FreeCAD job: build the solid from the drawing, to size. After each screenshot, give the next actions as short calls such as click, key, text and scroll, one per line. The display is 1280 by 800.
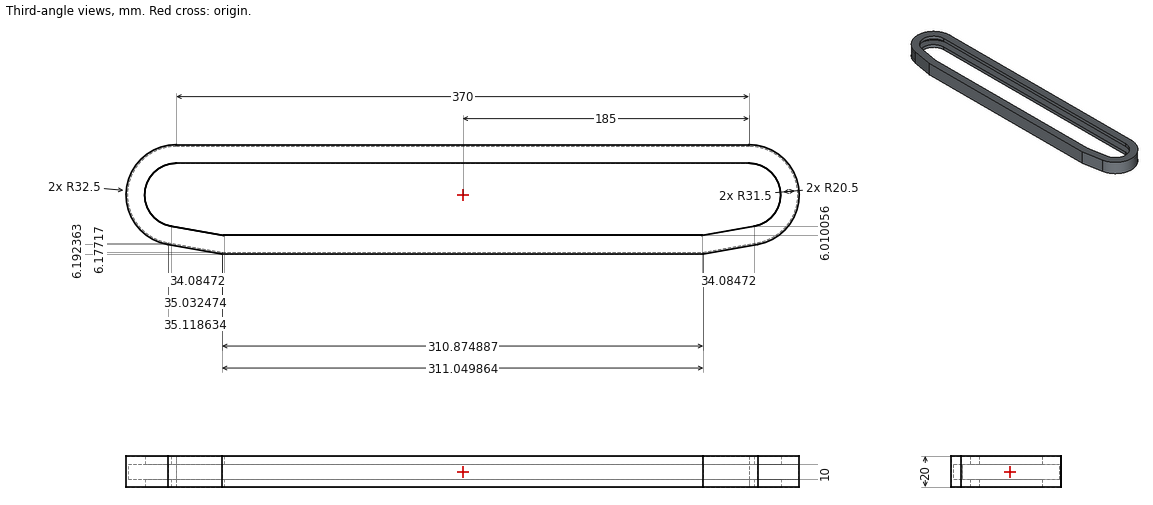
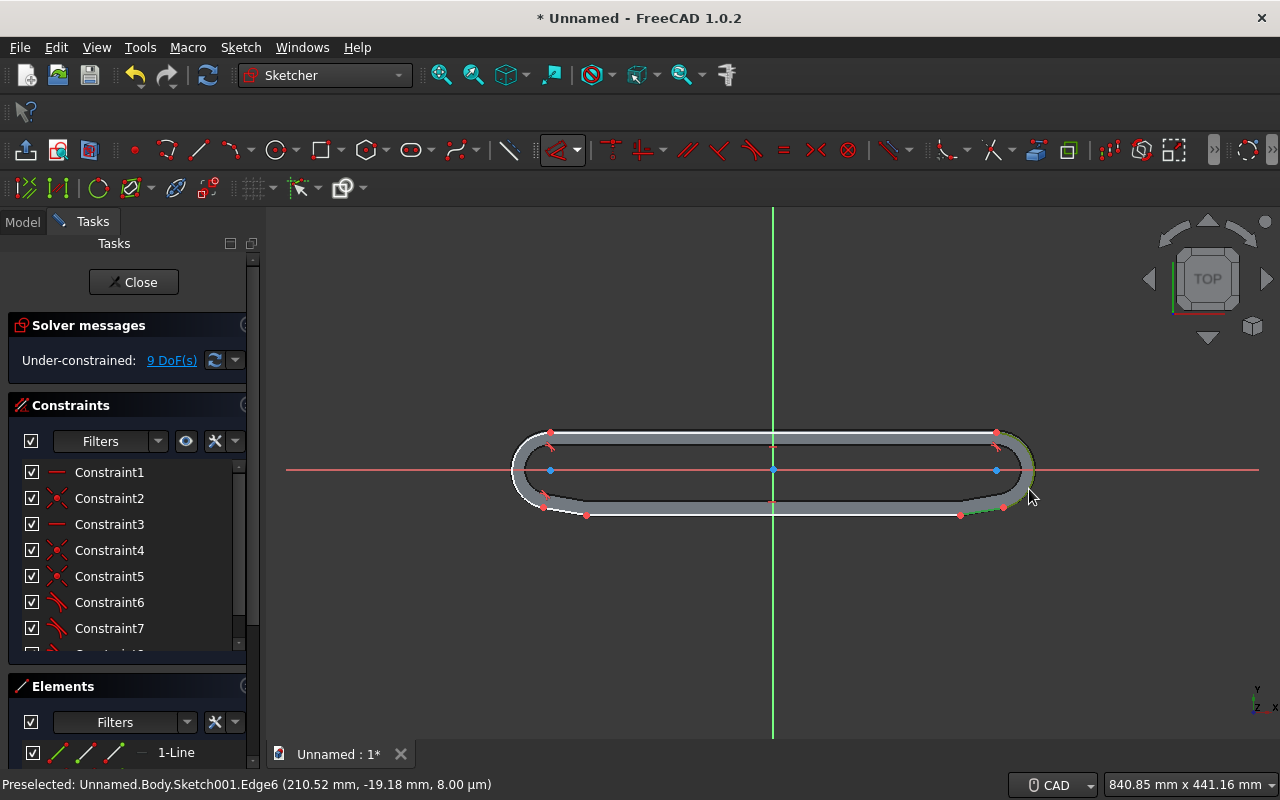
click(752, 150)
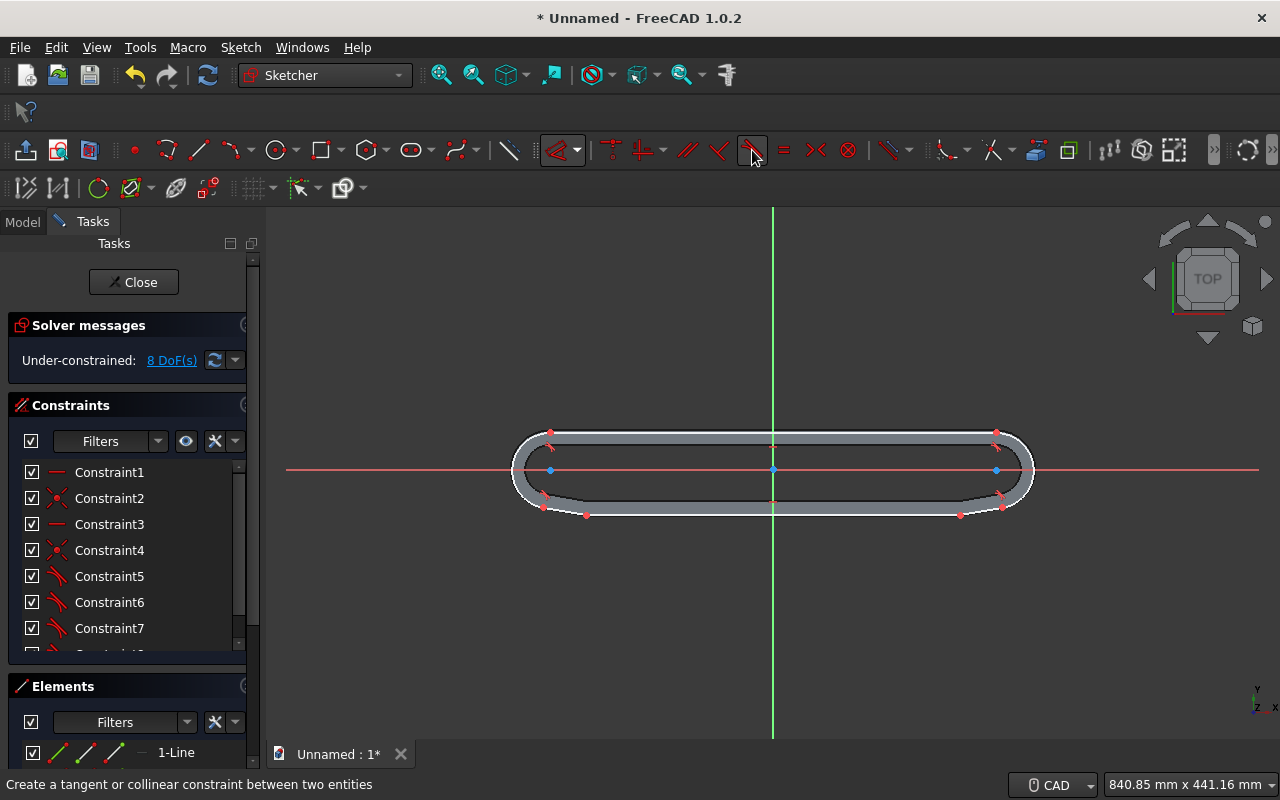
click(521, 447)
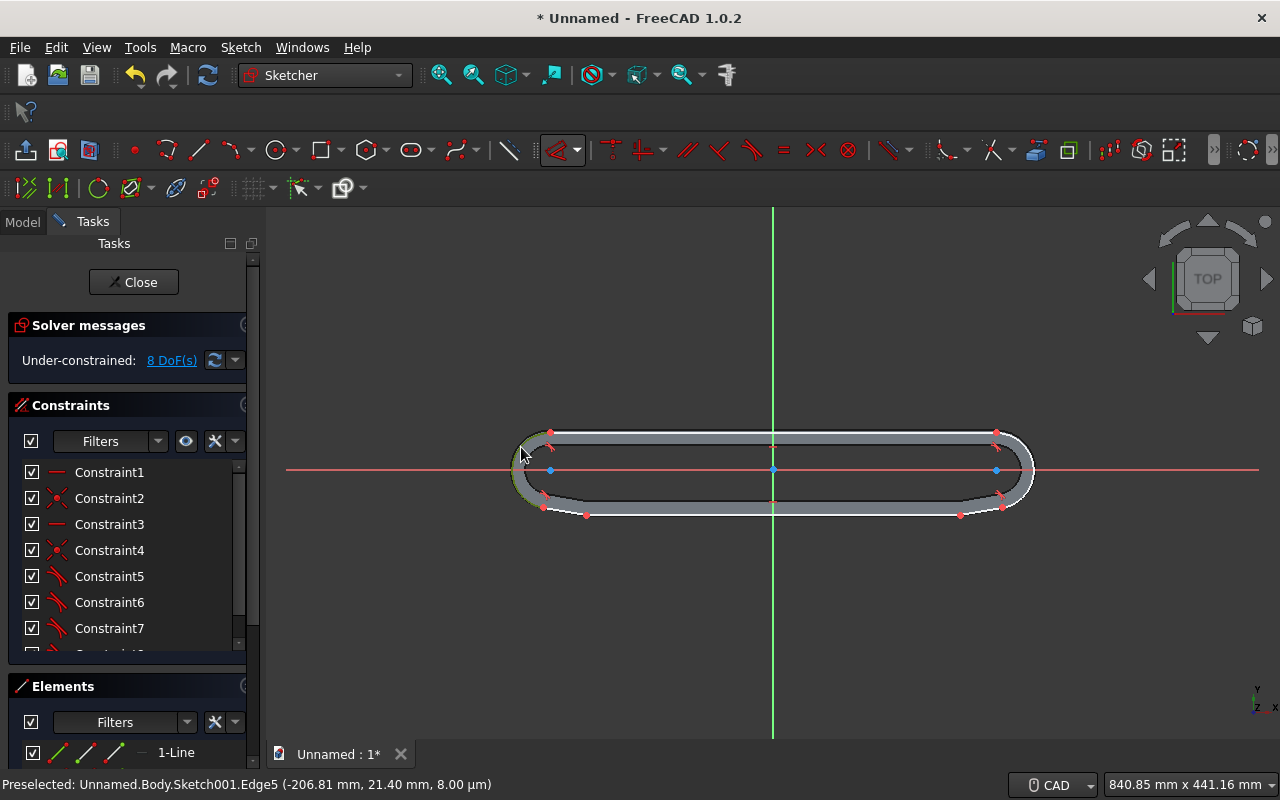
click(1029, 489)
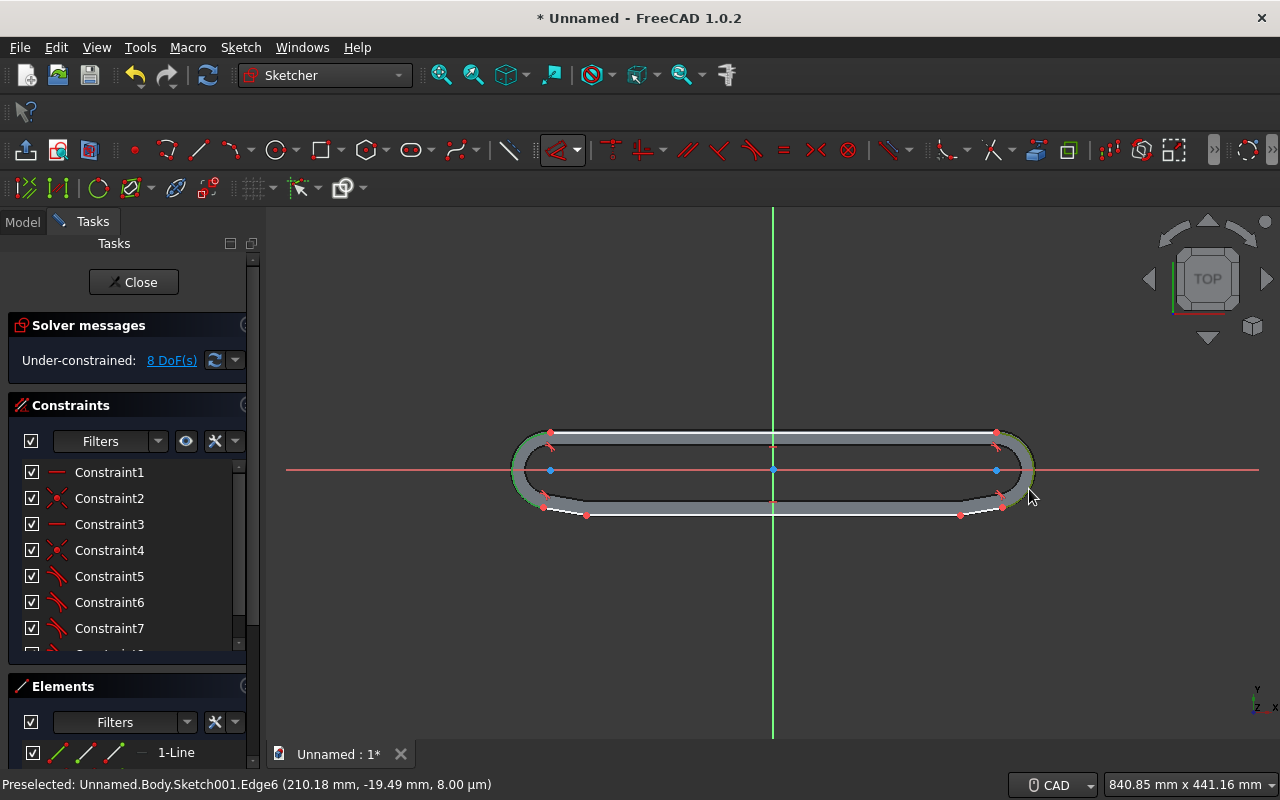
key(e)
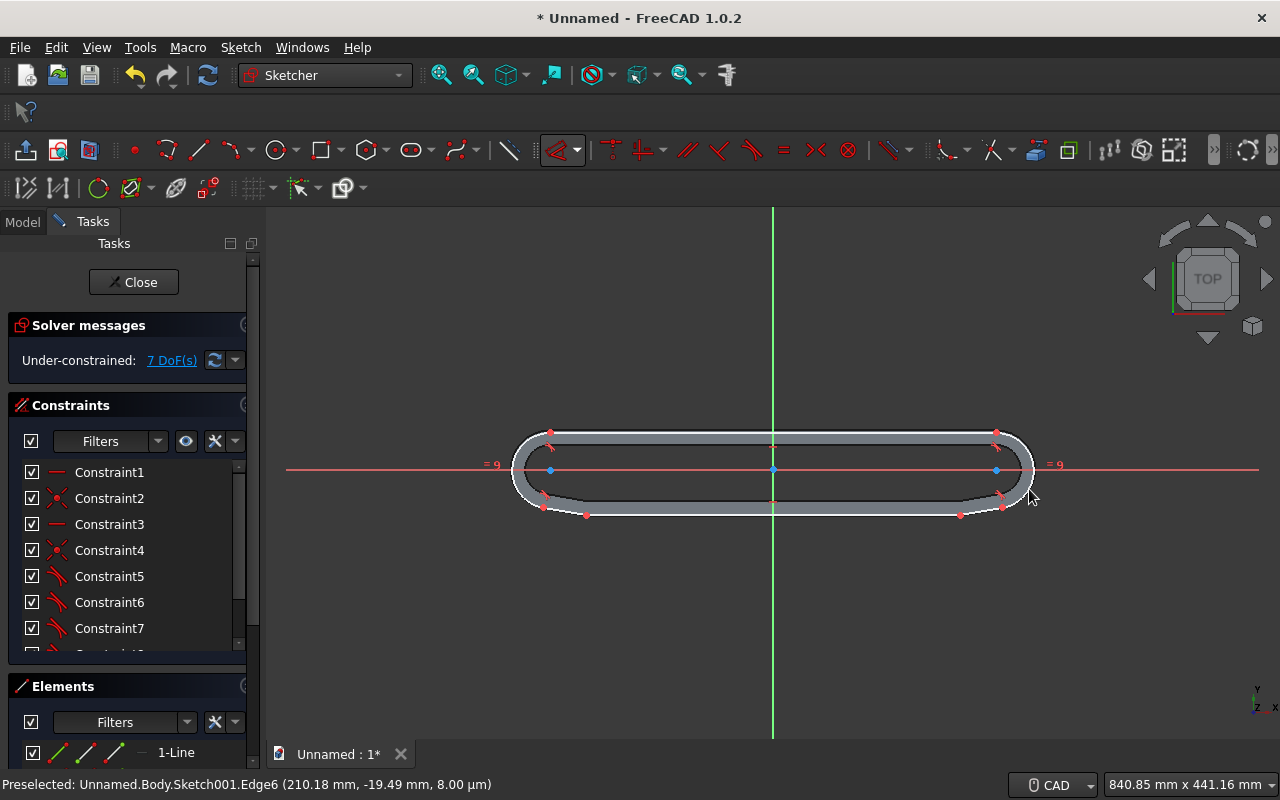
click(550, 471)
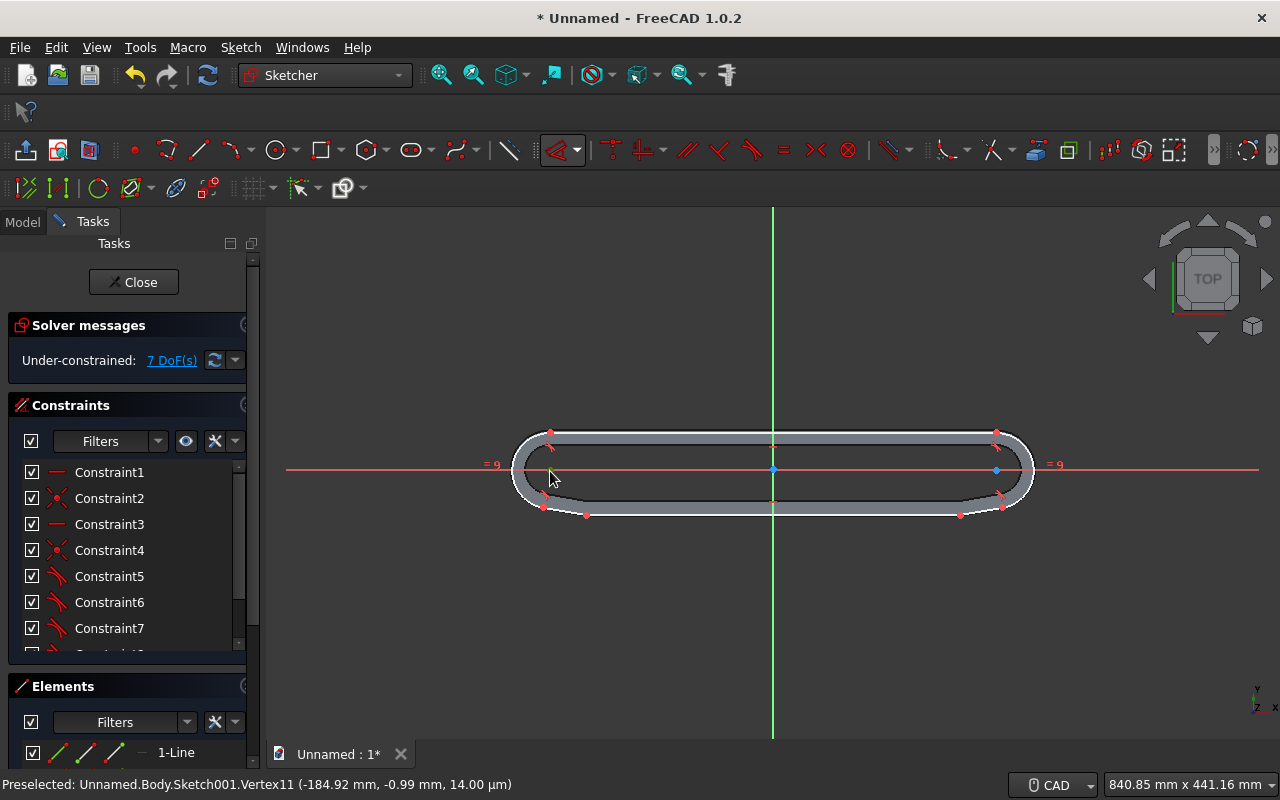
click(353, 470)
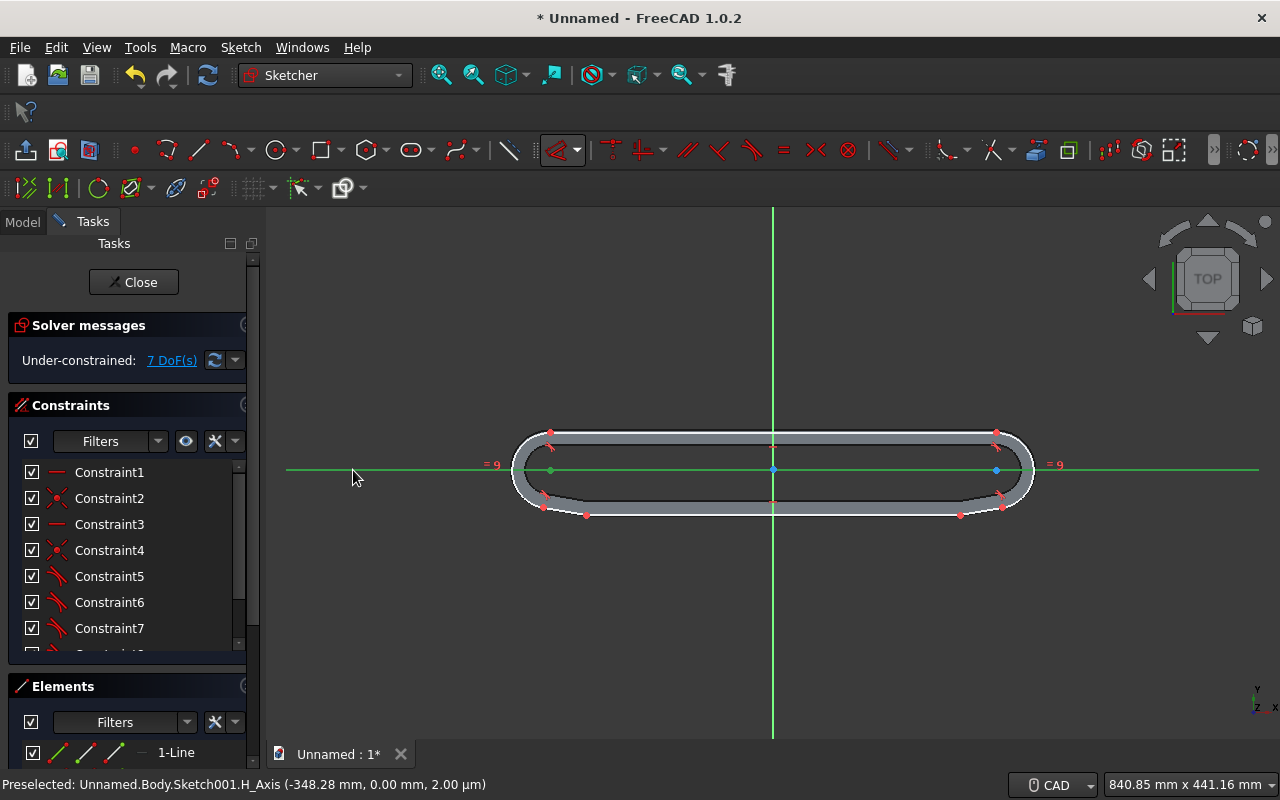
click(612, 150)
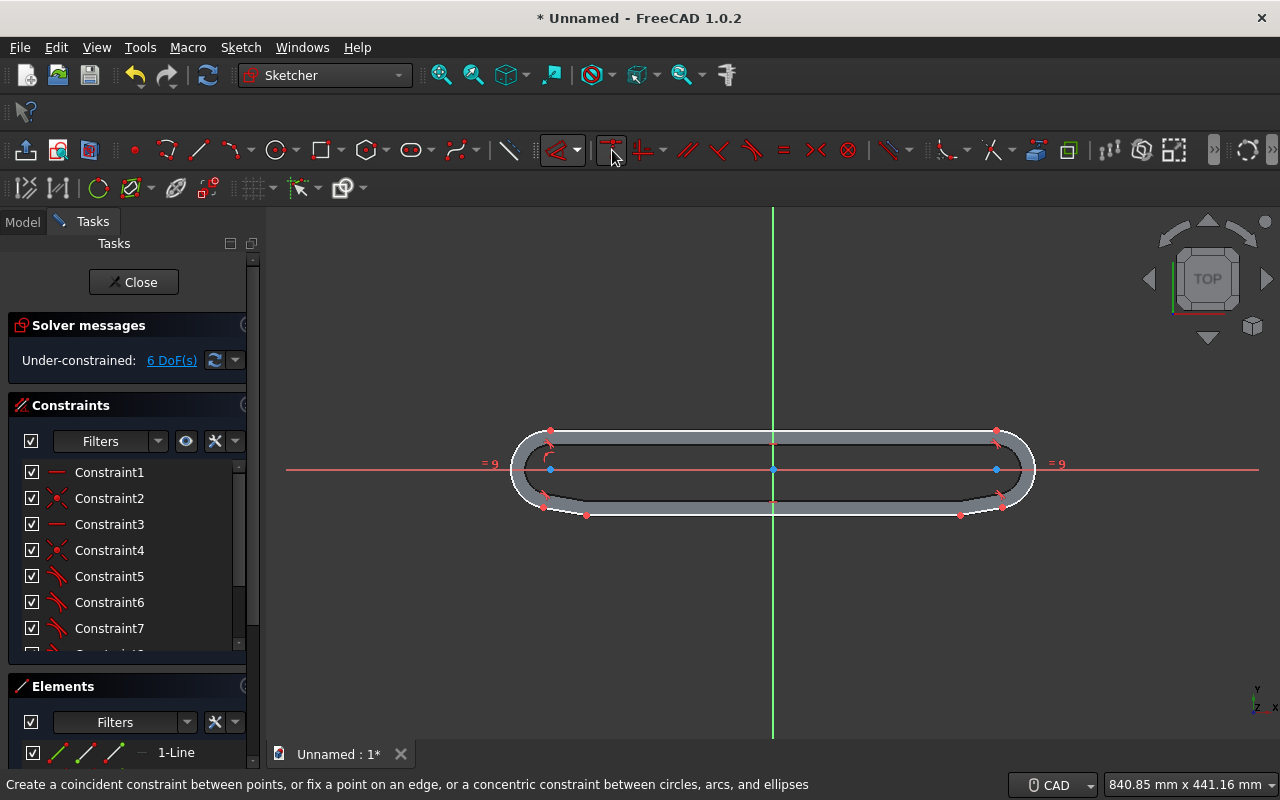
click(520, 445)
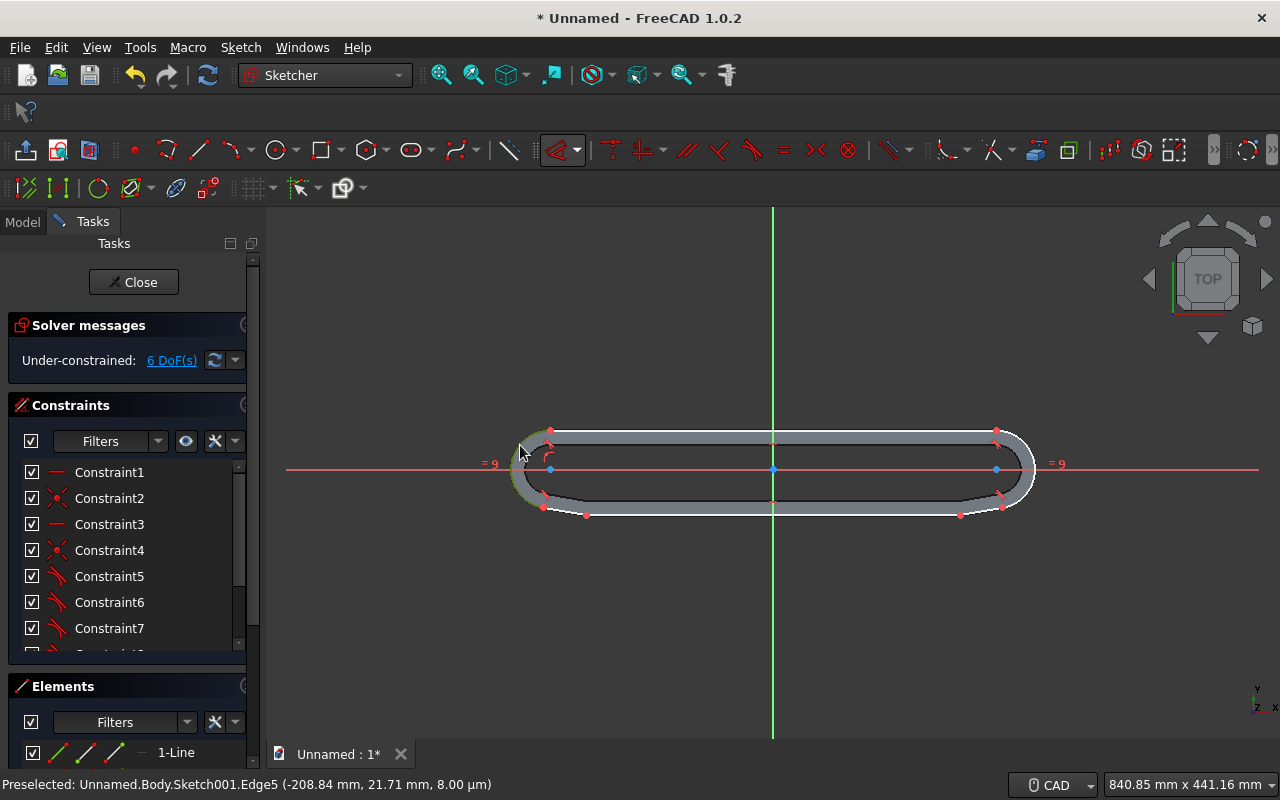
key(k)
key(r)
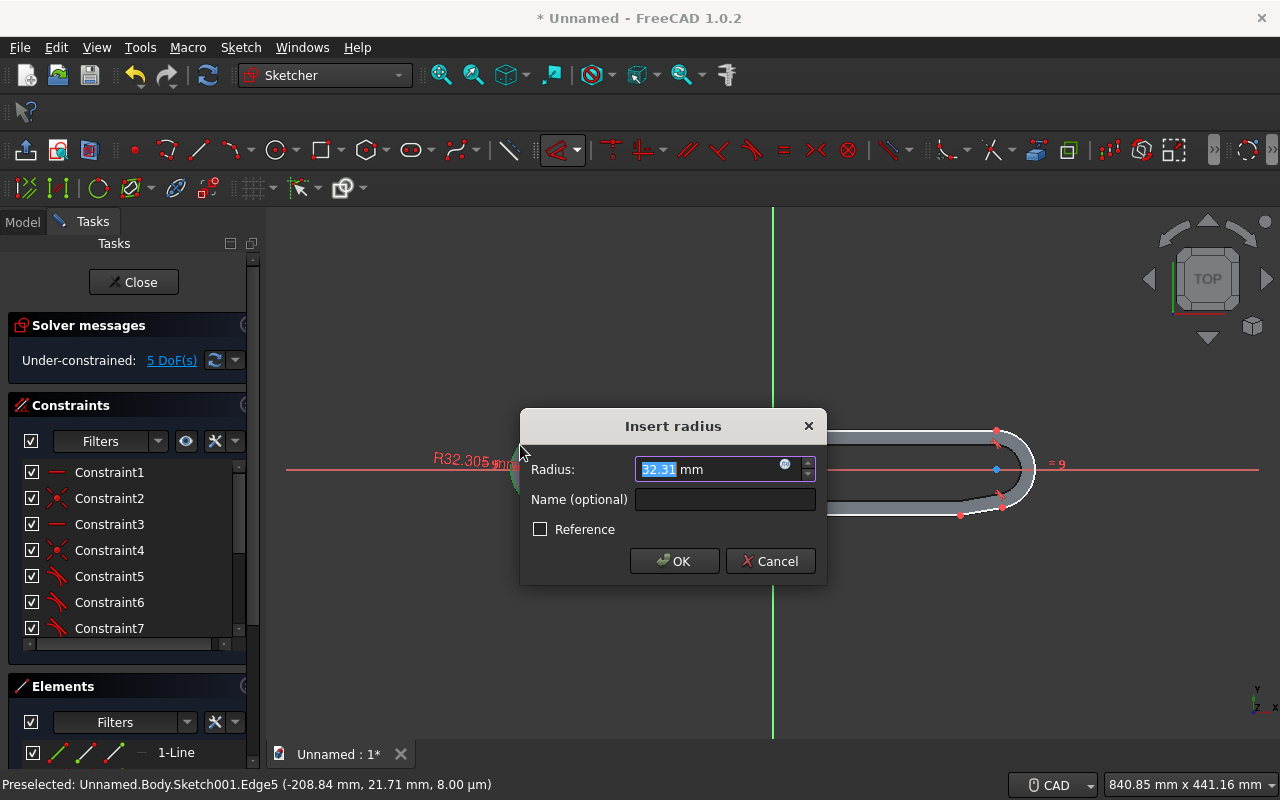
text(31.5)
key(Return)